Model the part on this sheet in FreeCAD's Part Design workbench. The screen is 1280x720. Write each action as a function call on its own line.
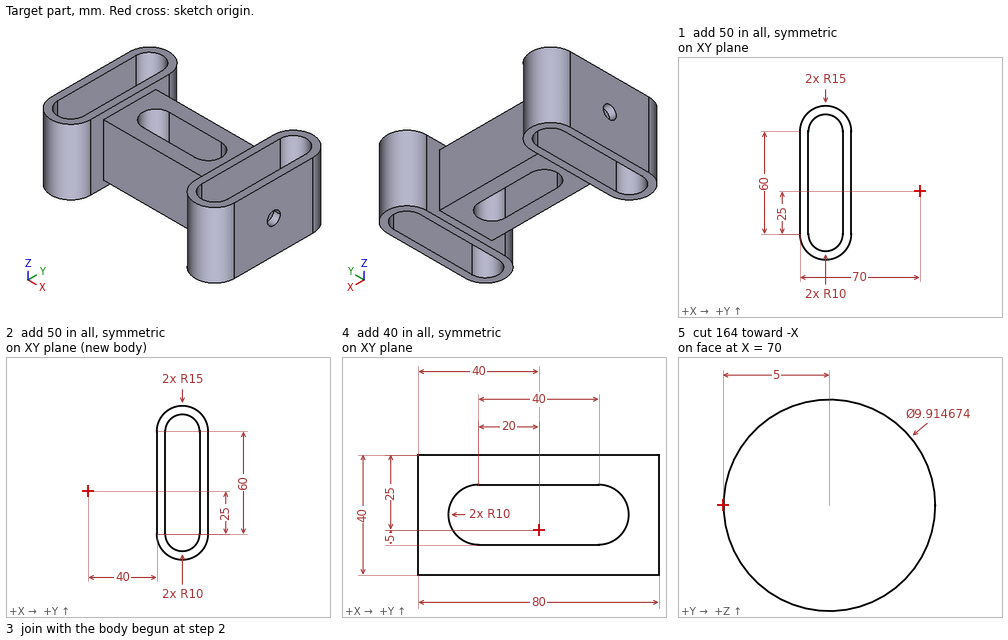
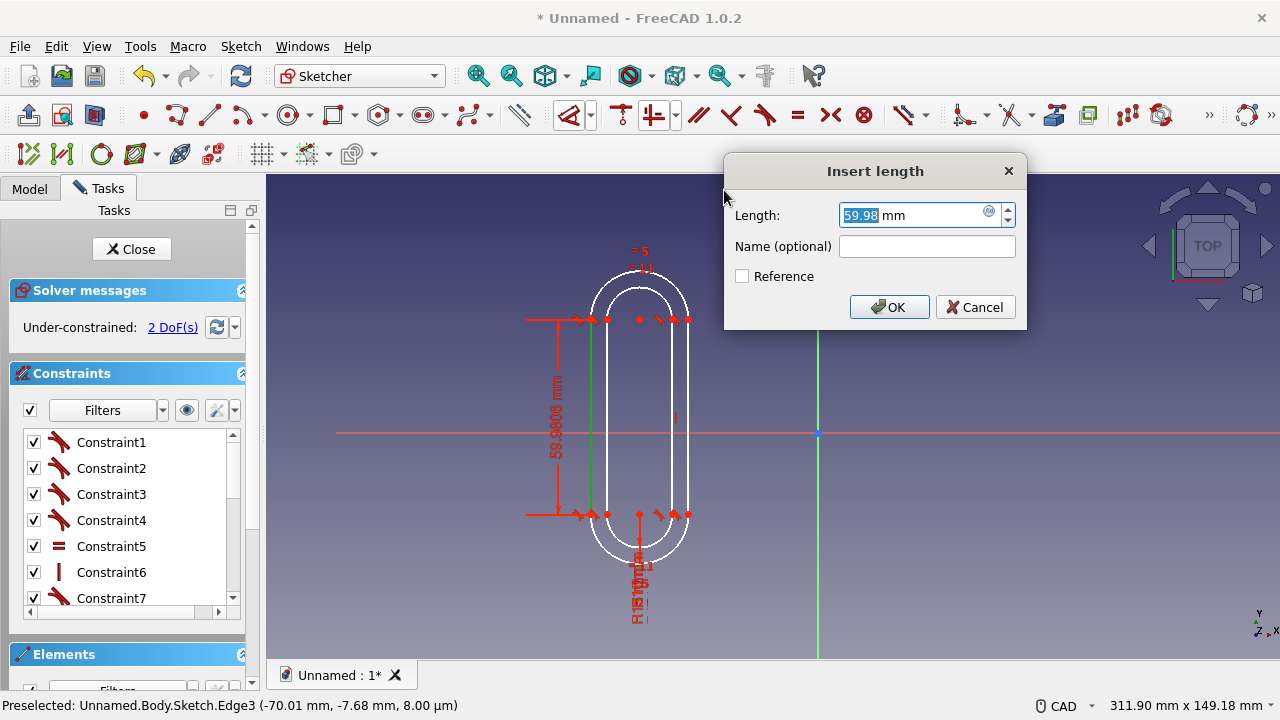
text(60)
key(Return)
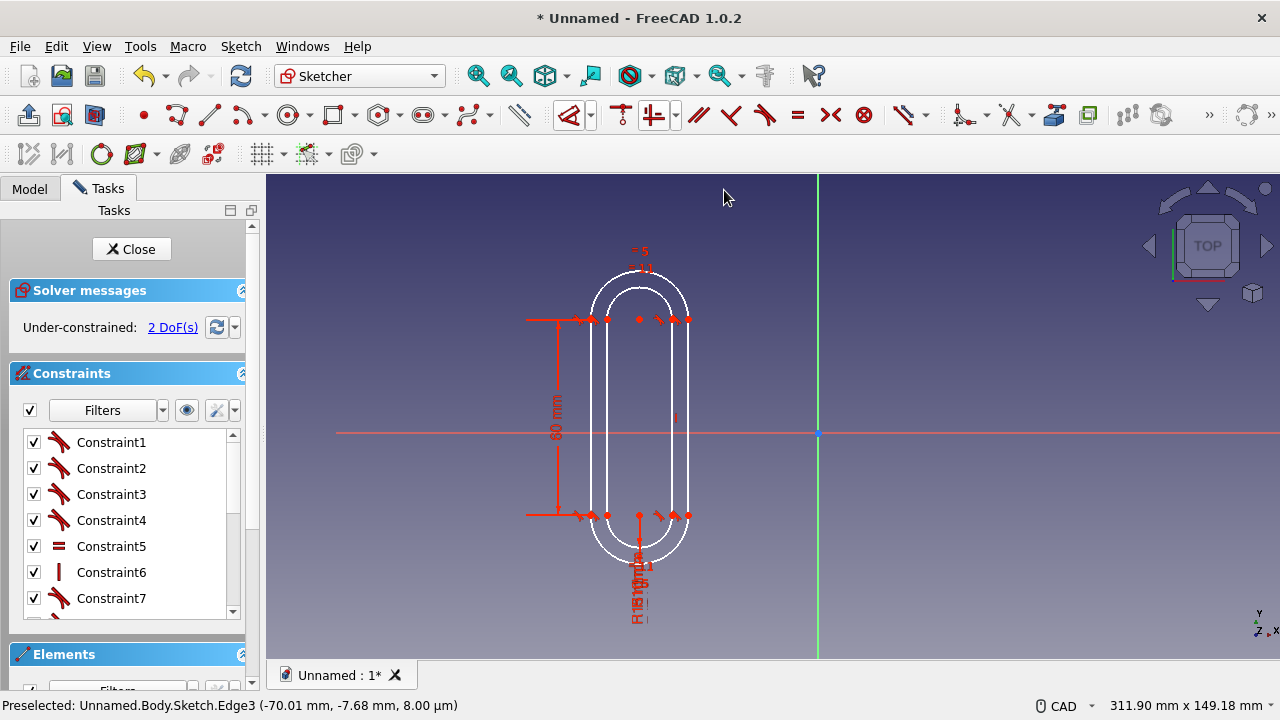
click(591, 515)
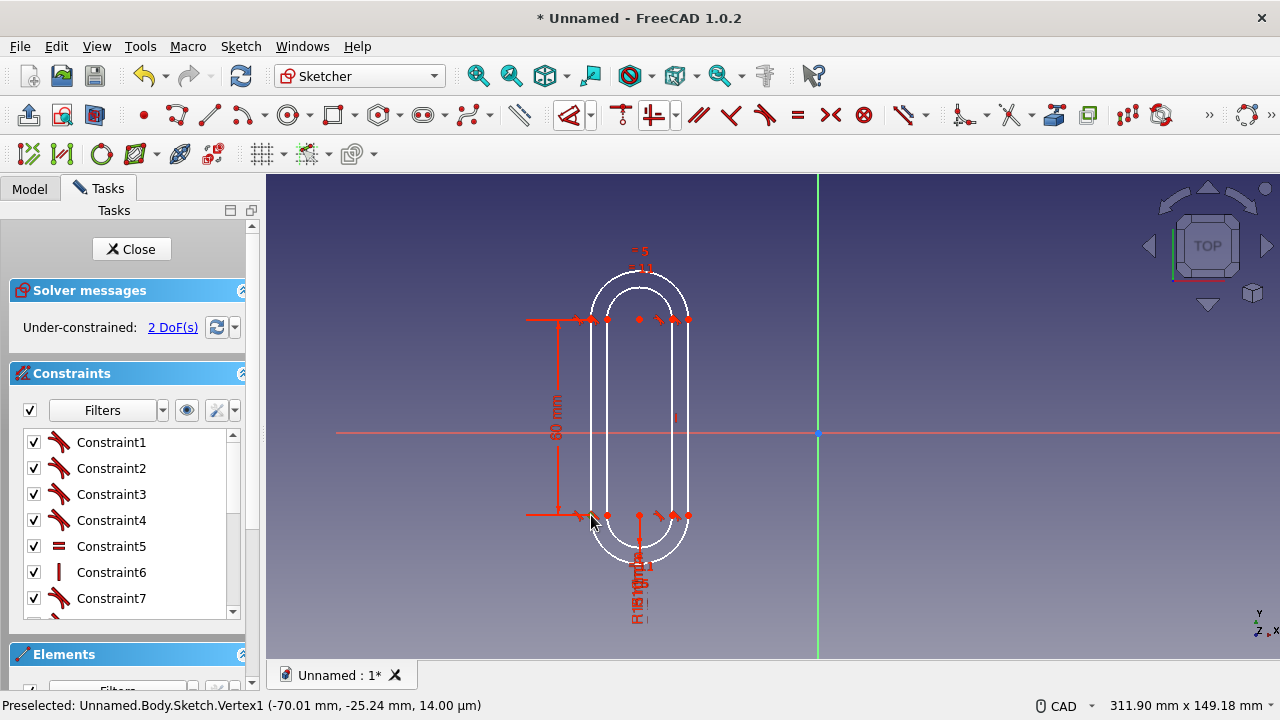
click(590, 116)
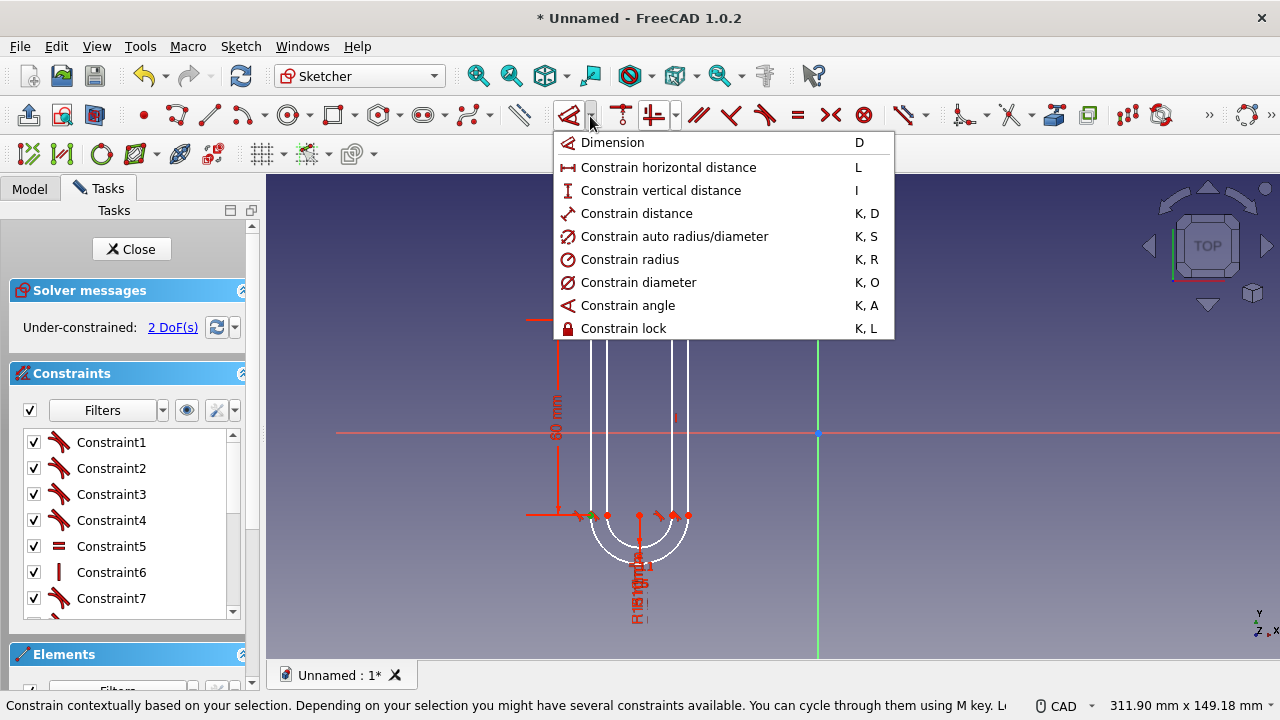
click(724, 168)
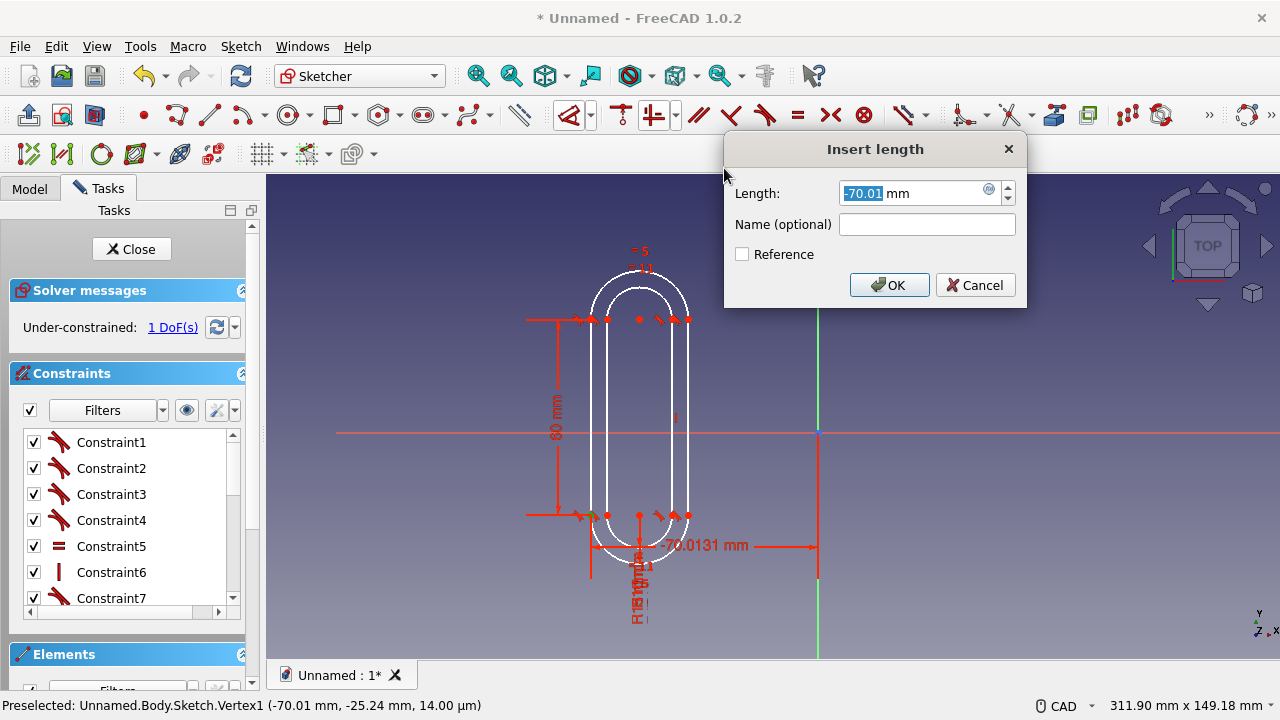
text(-70)
key(Return)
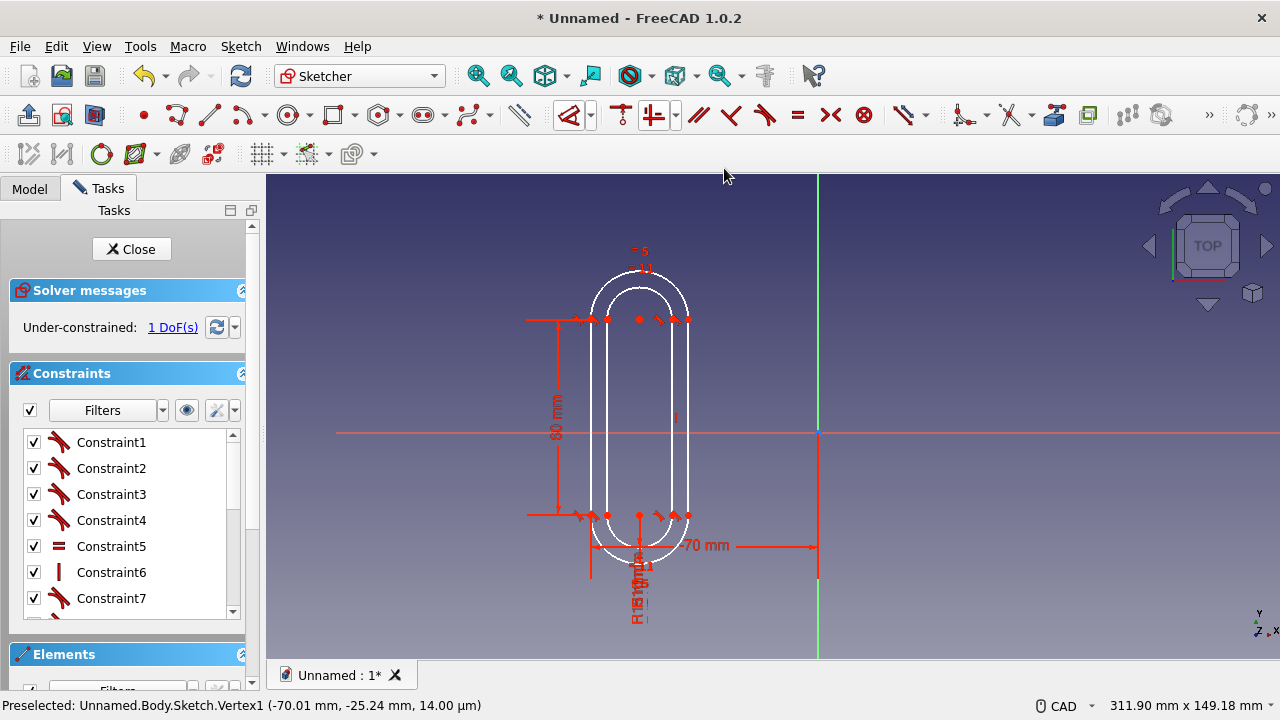
click(591, 515)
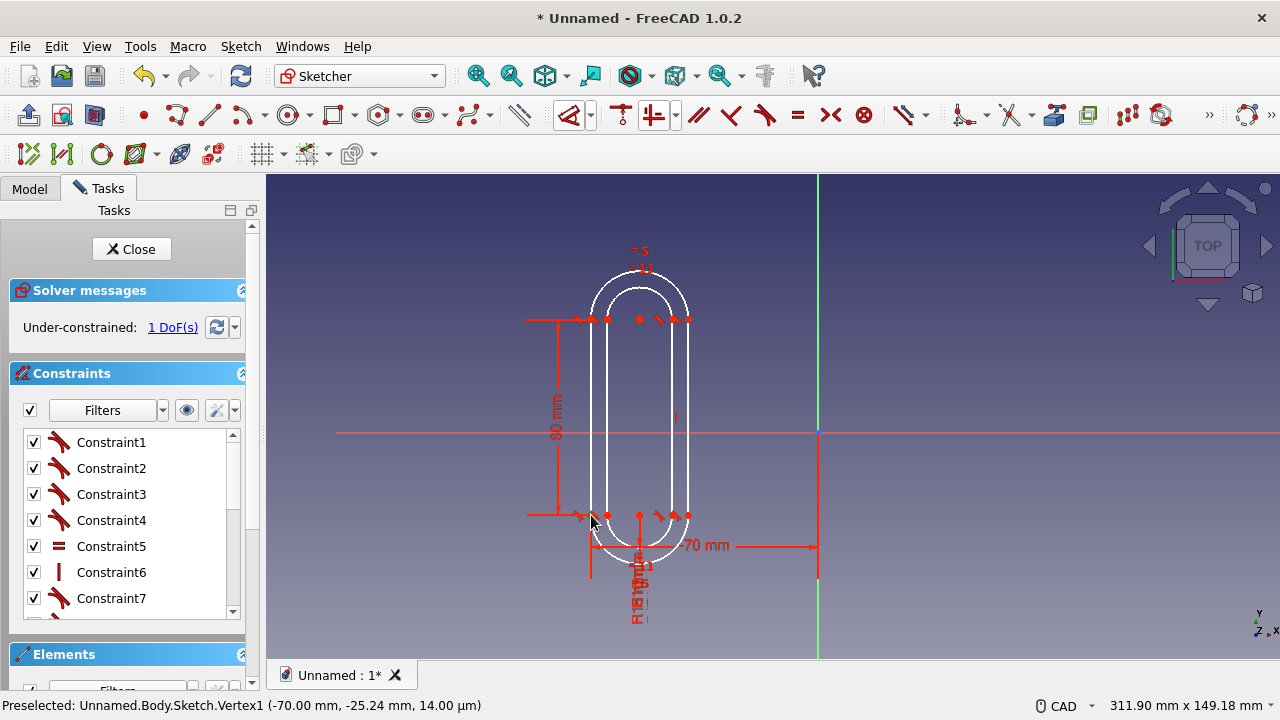
click(590, 116)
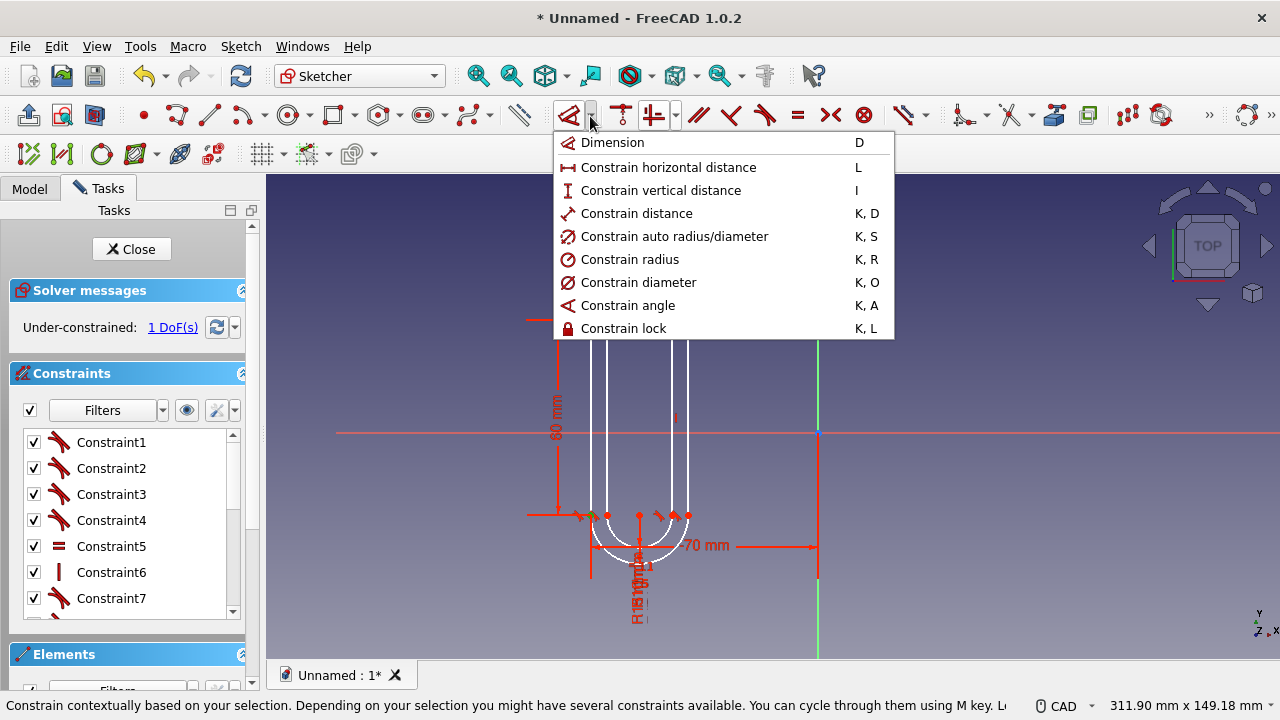
click(724, 190)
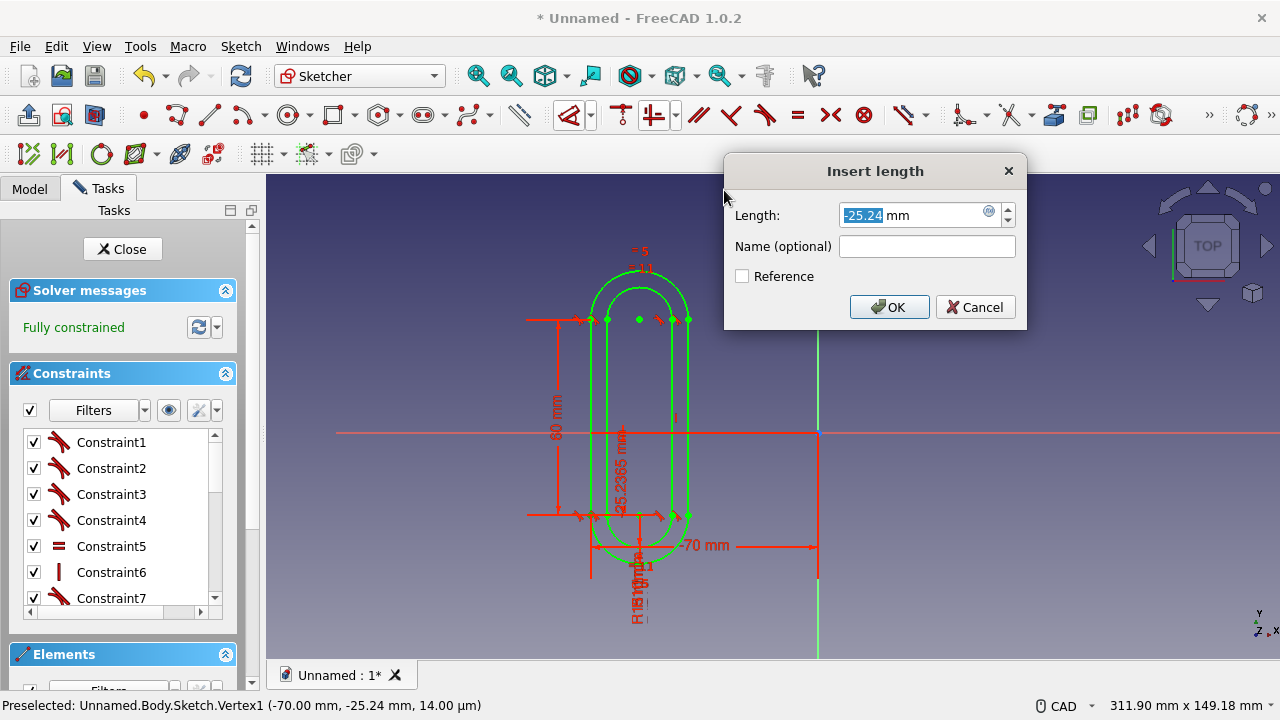
text(-25)
key(Return)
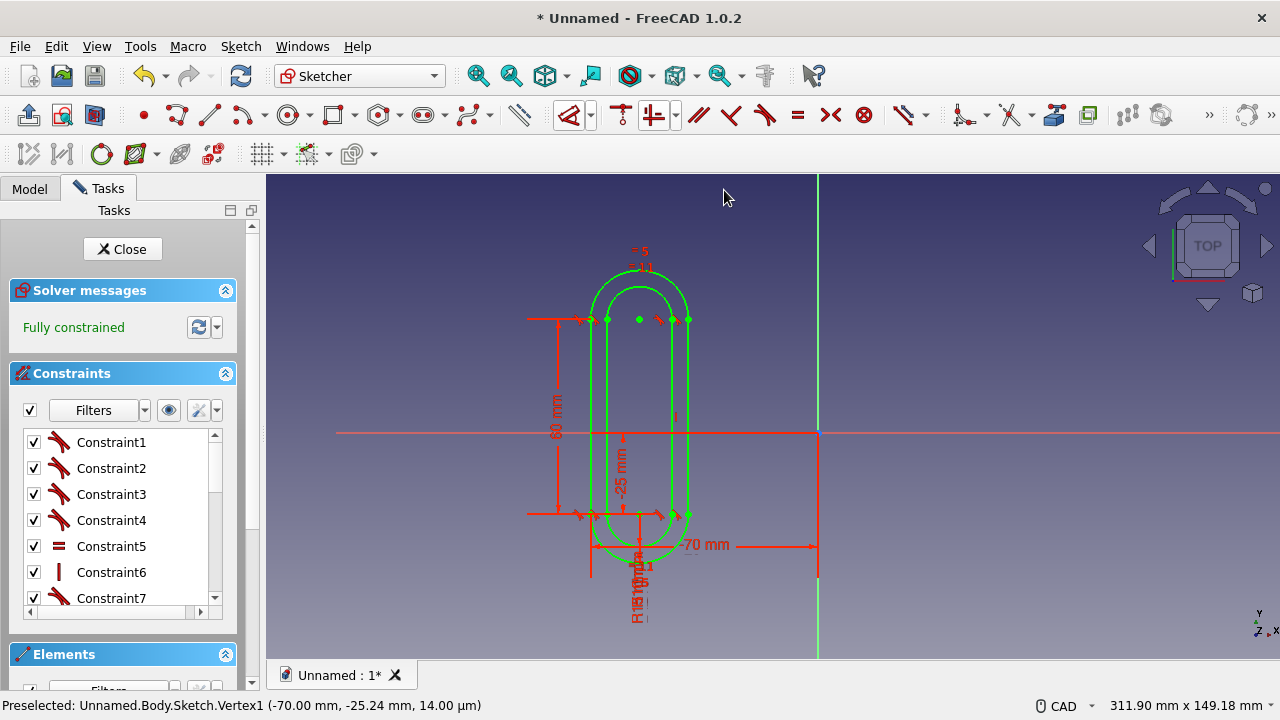
click(123, 249)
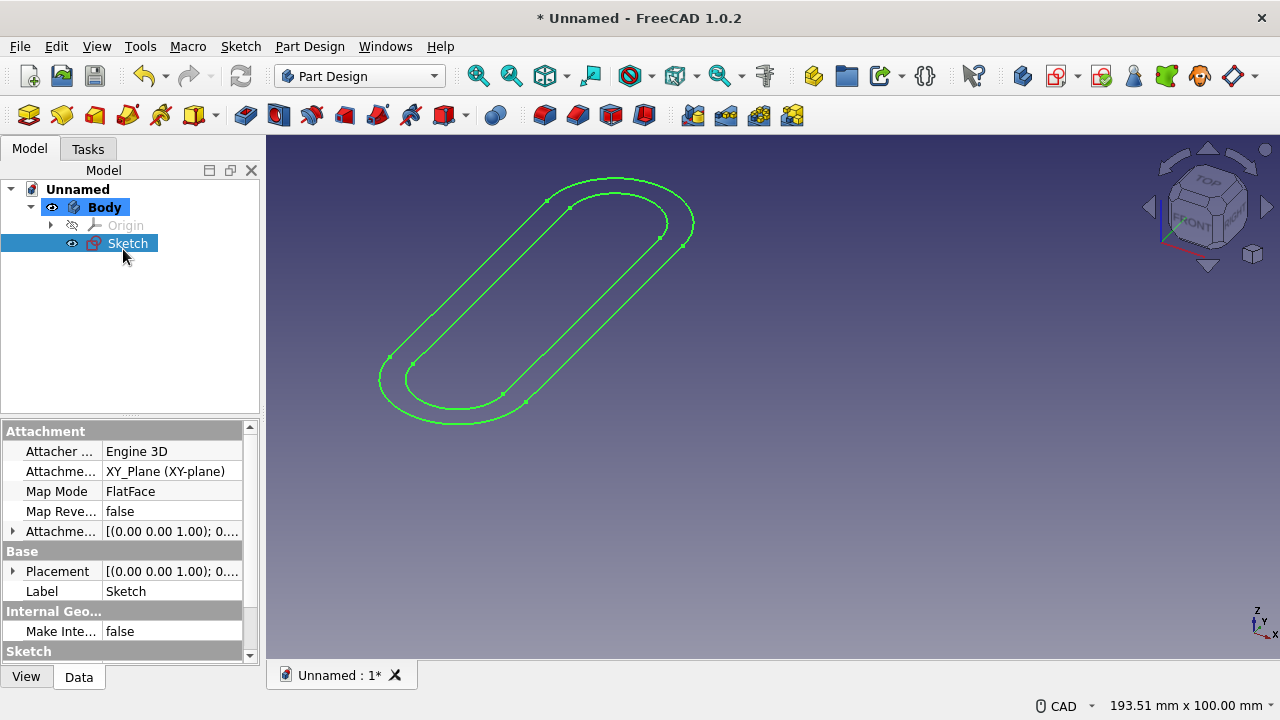
click(29, 116)